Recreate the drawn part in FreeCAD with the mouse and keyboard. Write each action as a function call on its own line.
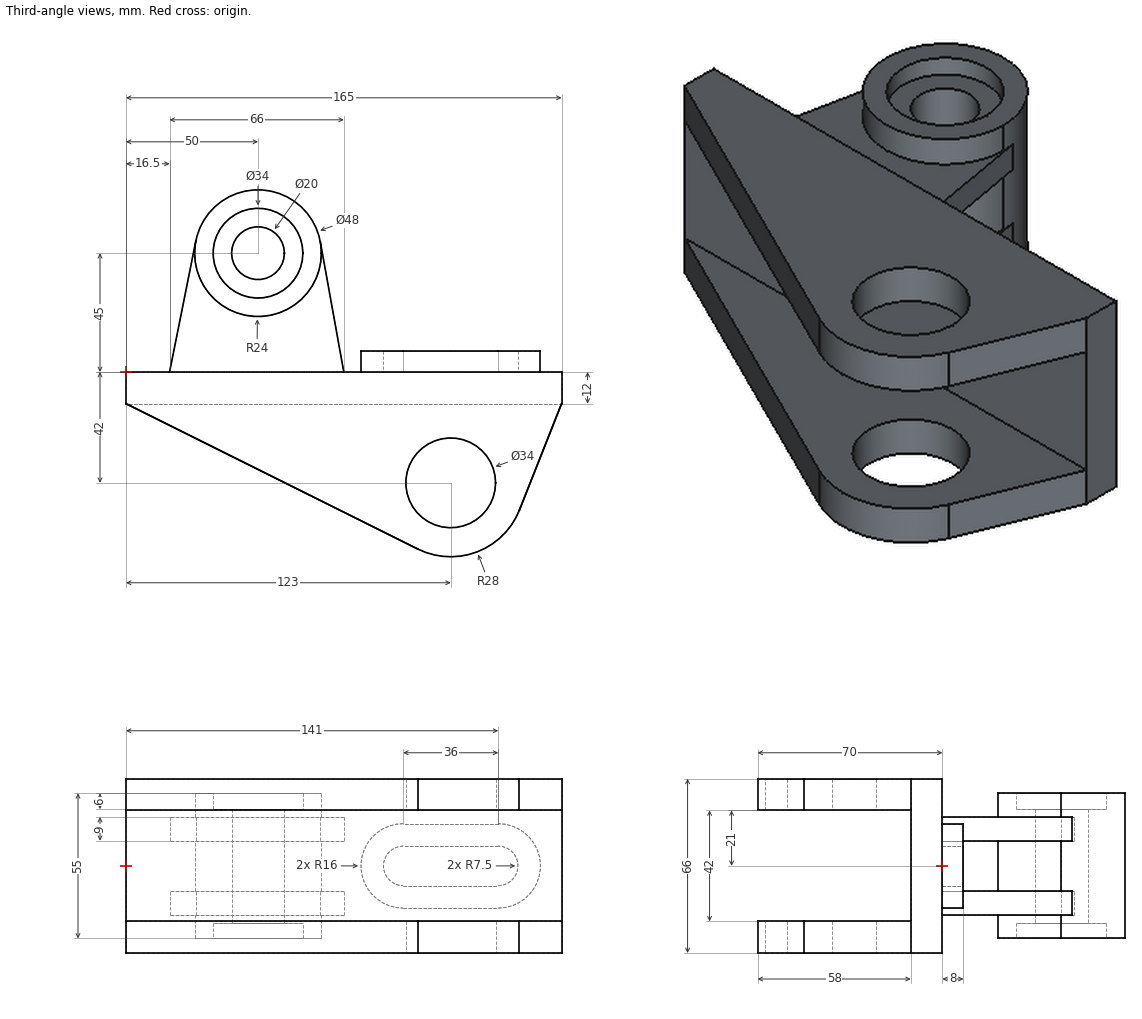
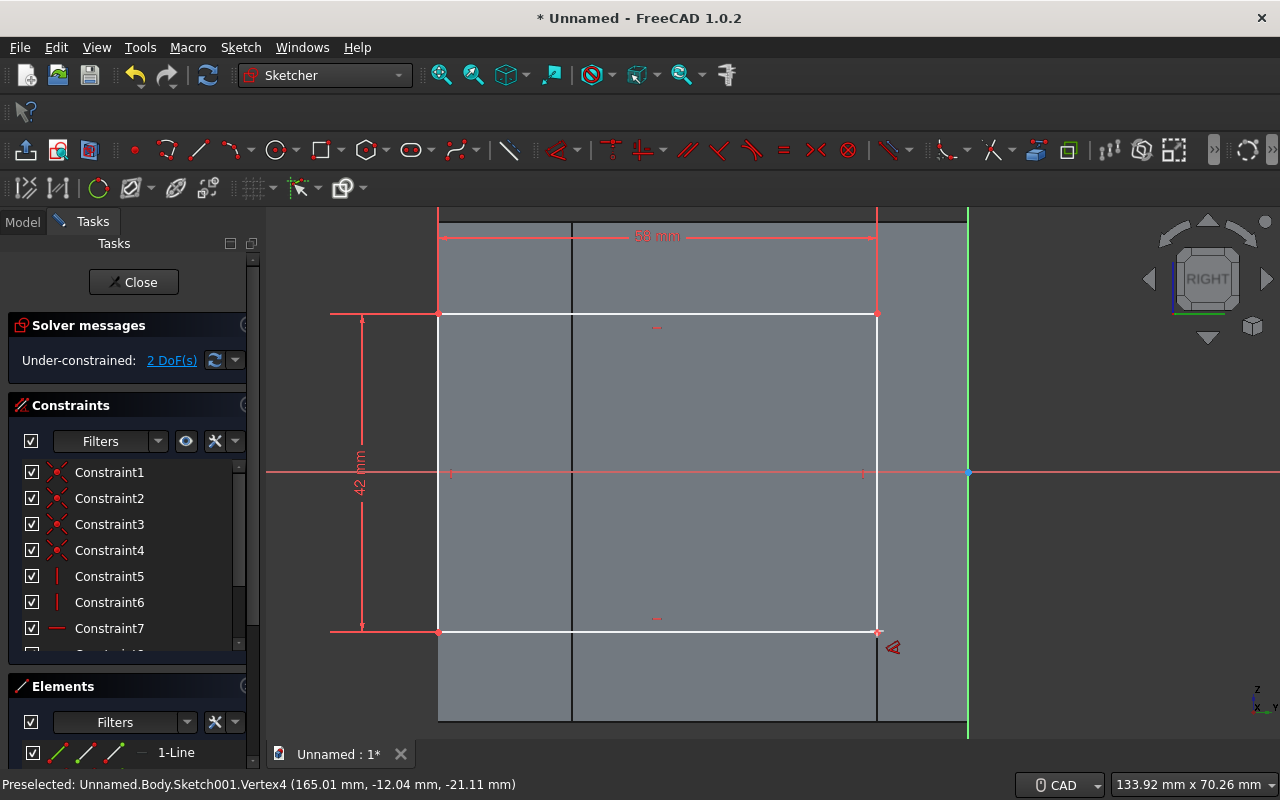
click(438, 314)
click(703, 280)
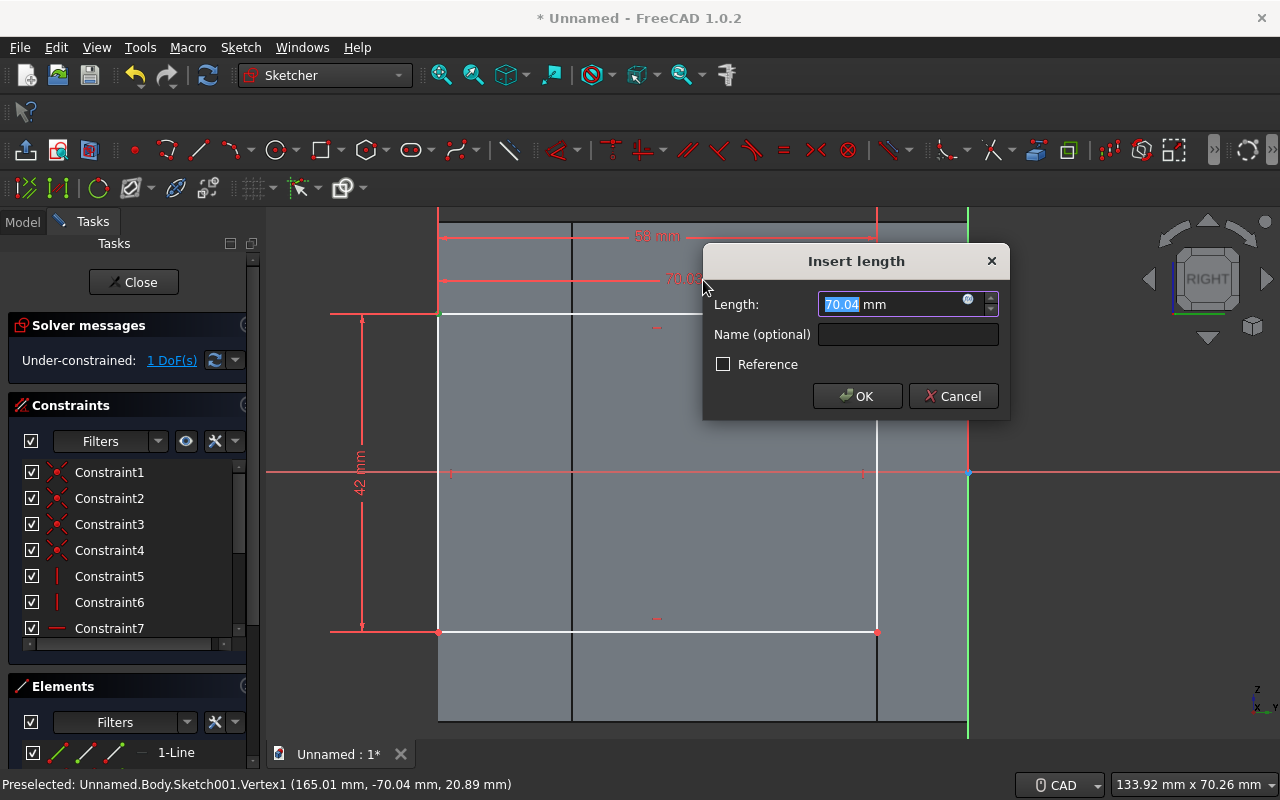
text(70)
key(Return)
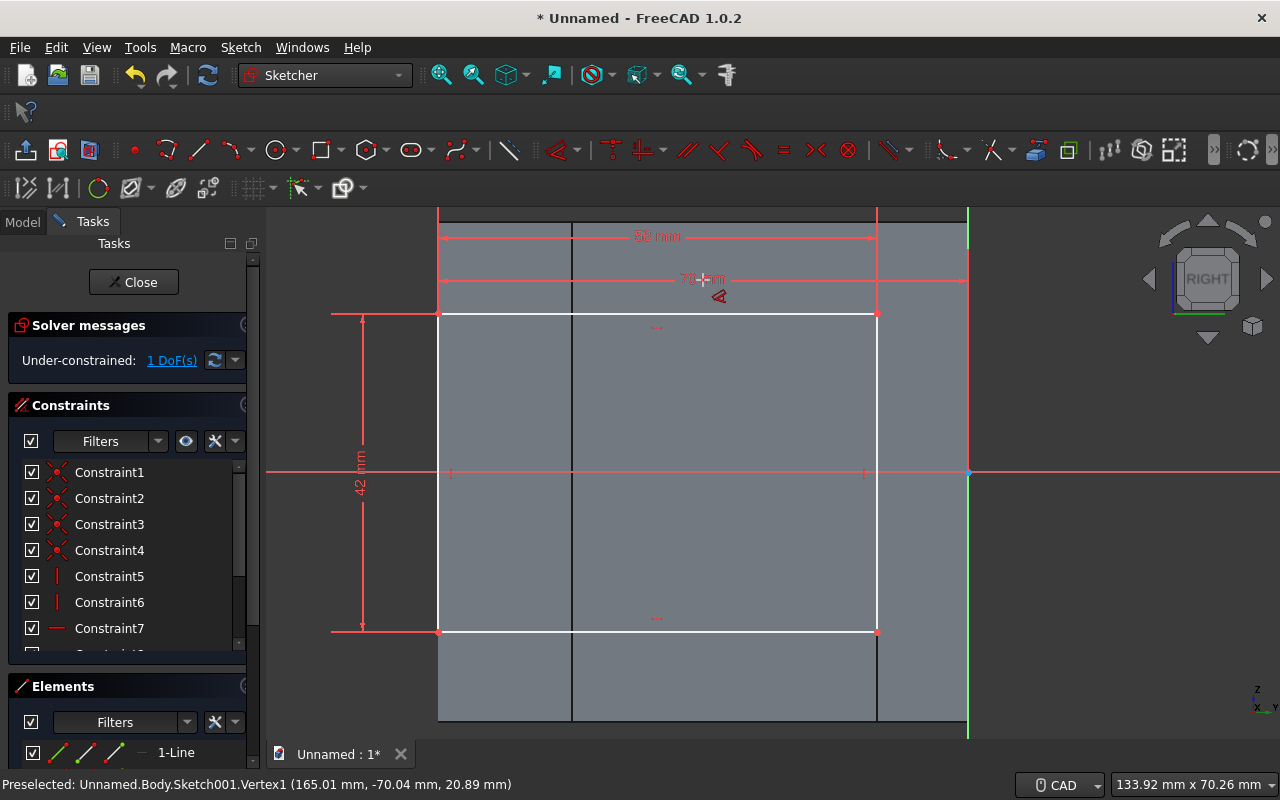
click(438, 314)
click(1002, 393)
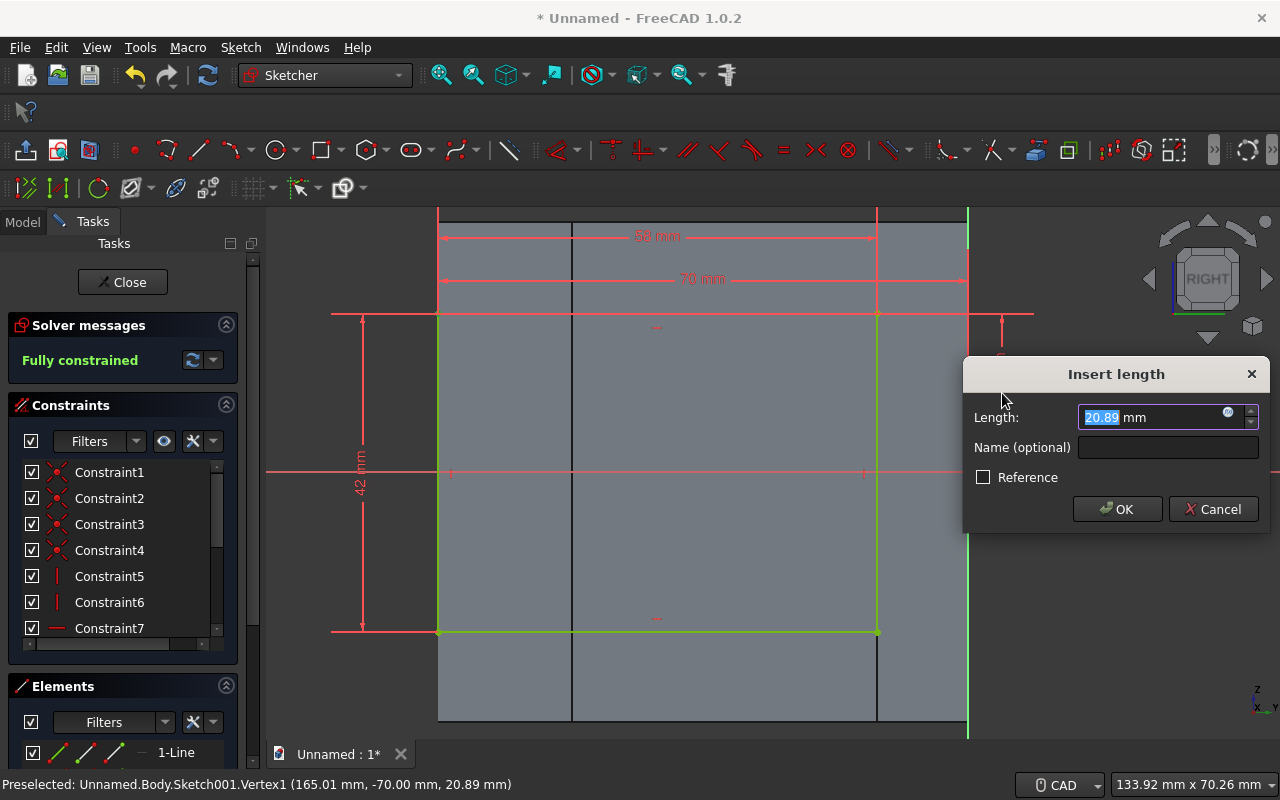
text(21)
key(Return)
key(Escape)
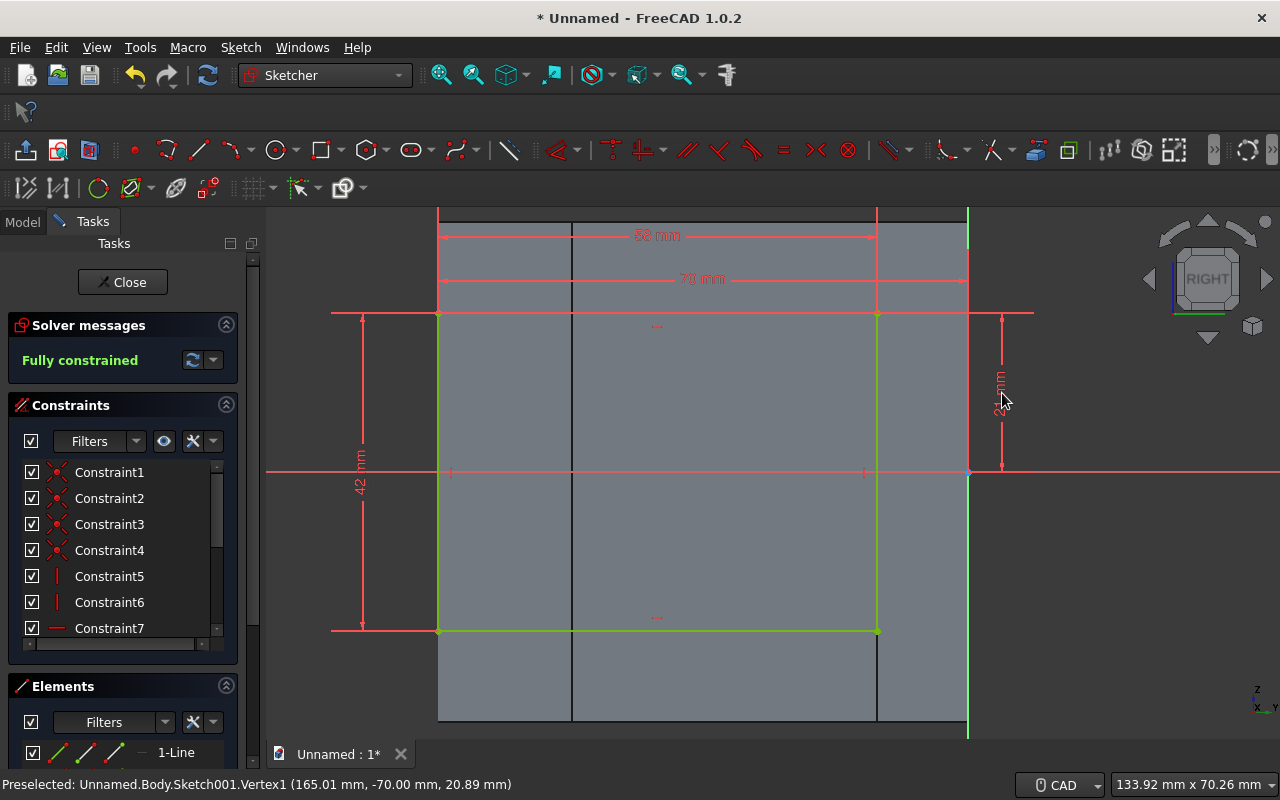
click(123, 282)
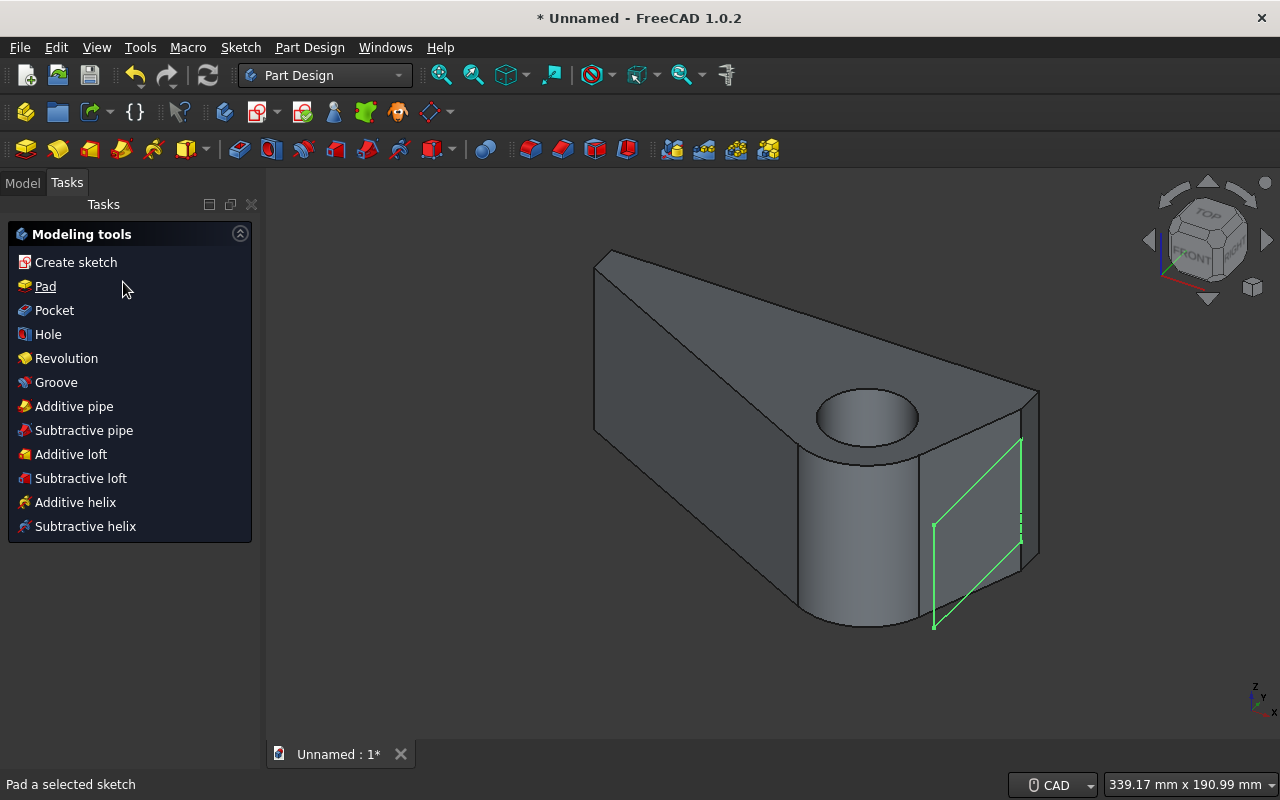
click(240, 150)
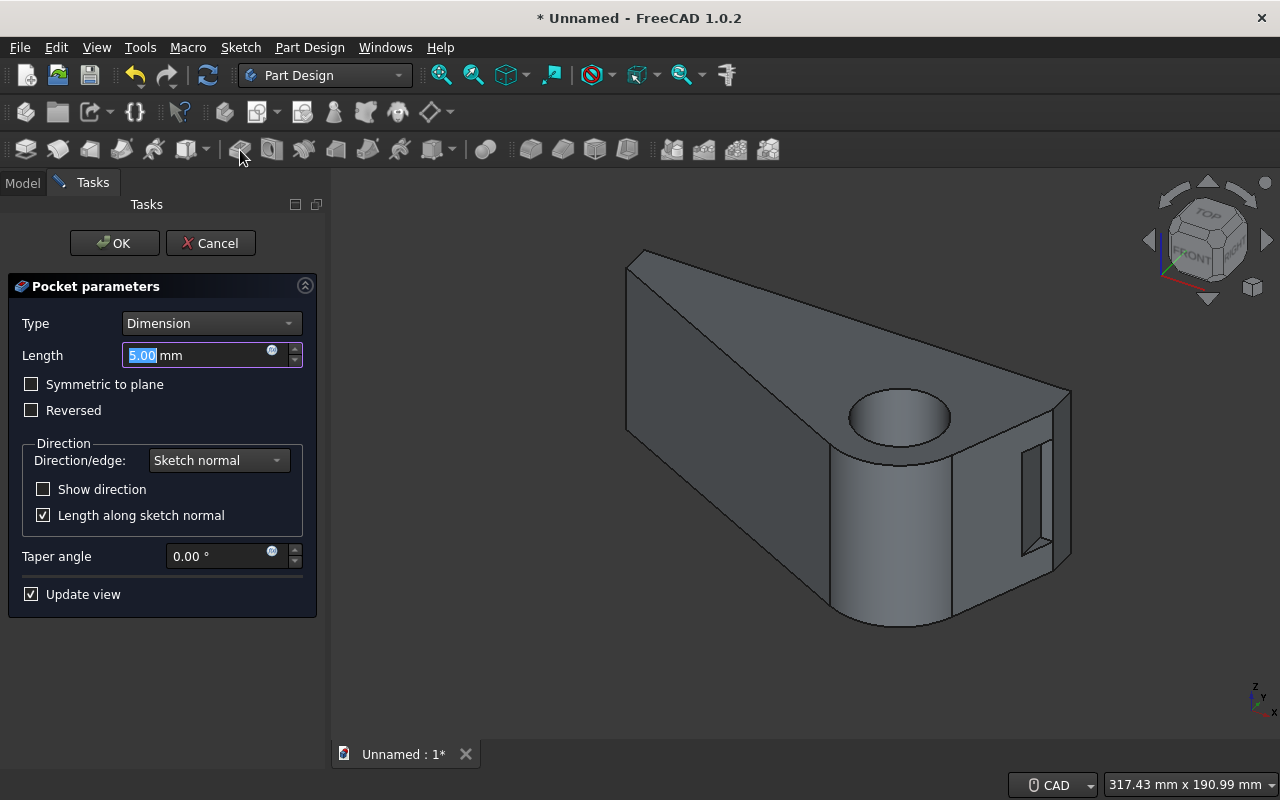
click(212, 324)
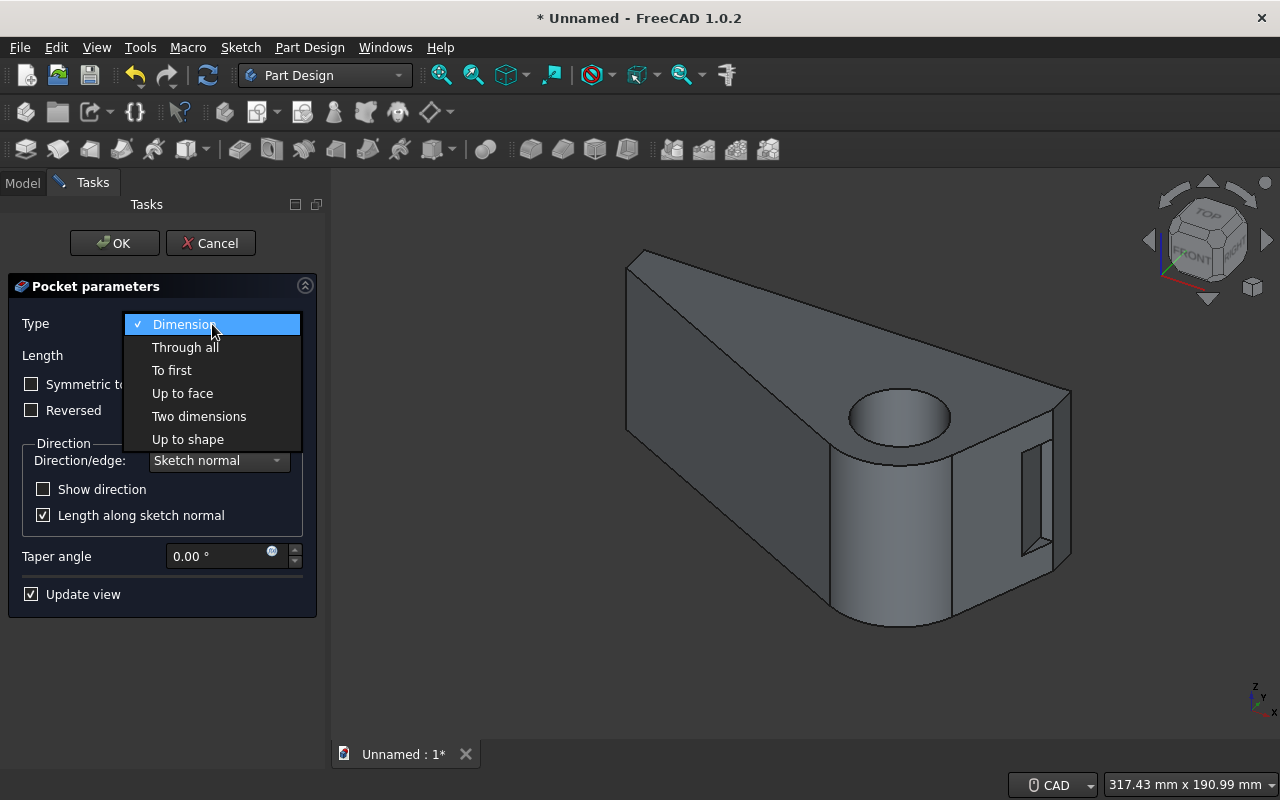
click(212, 348)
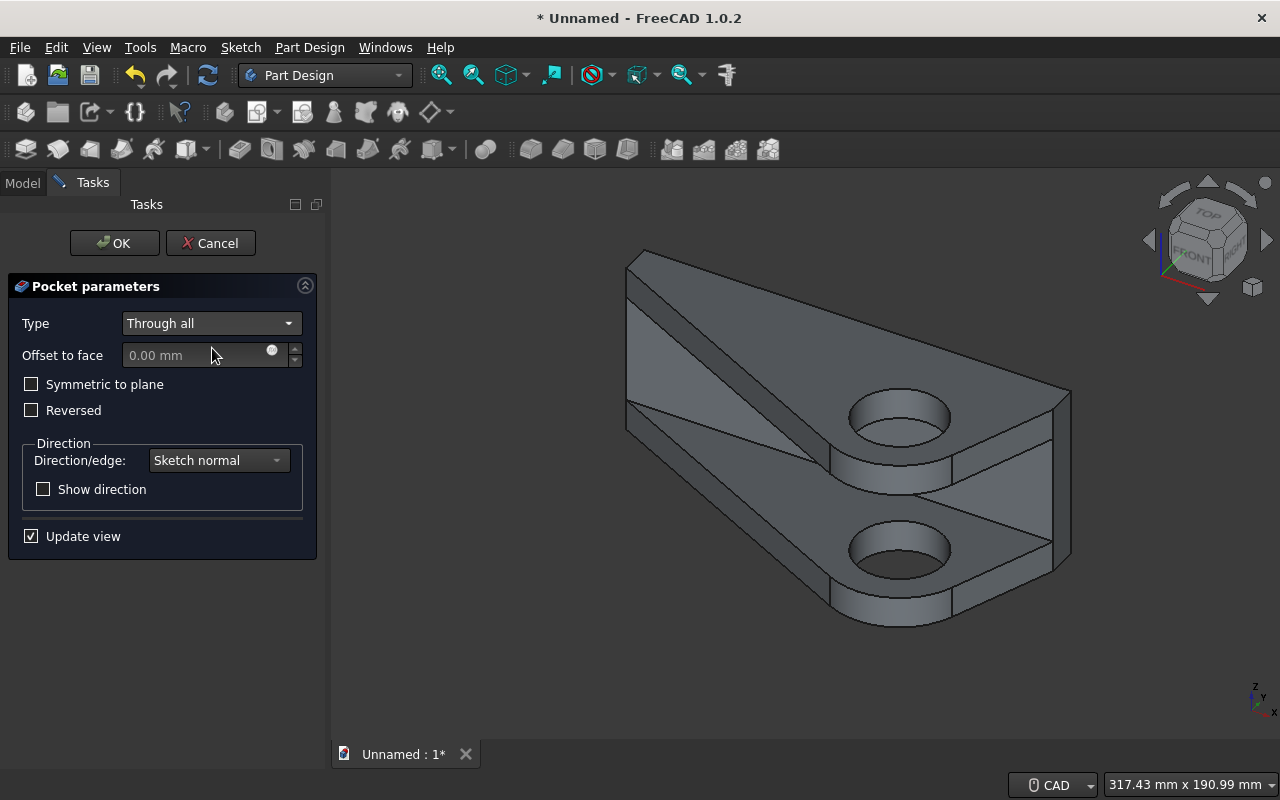
click(115, 243)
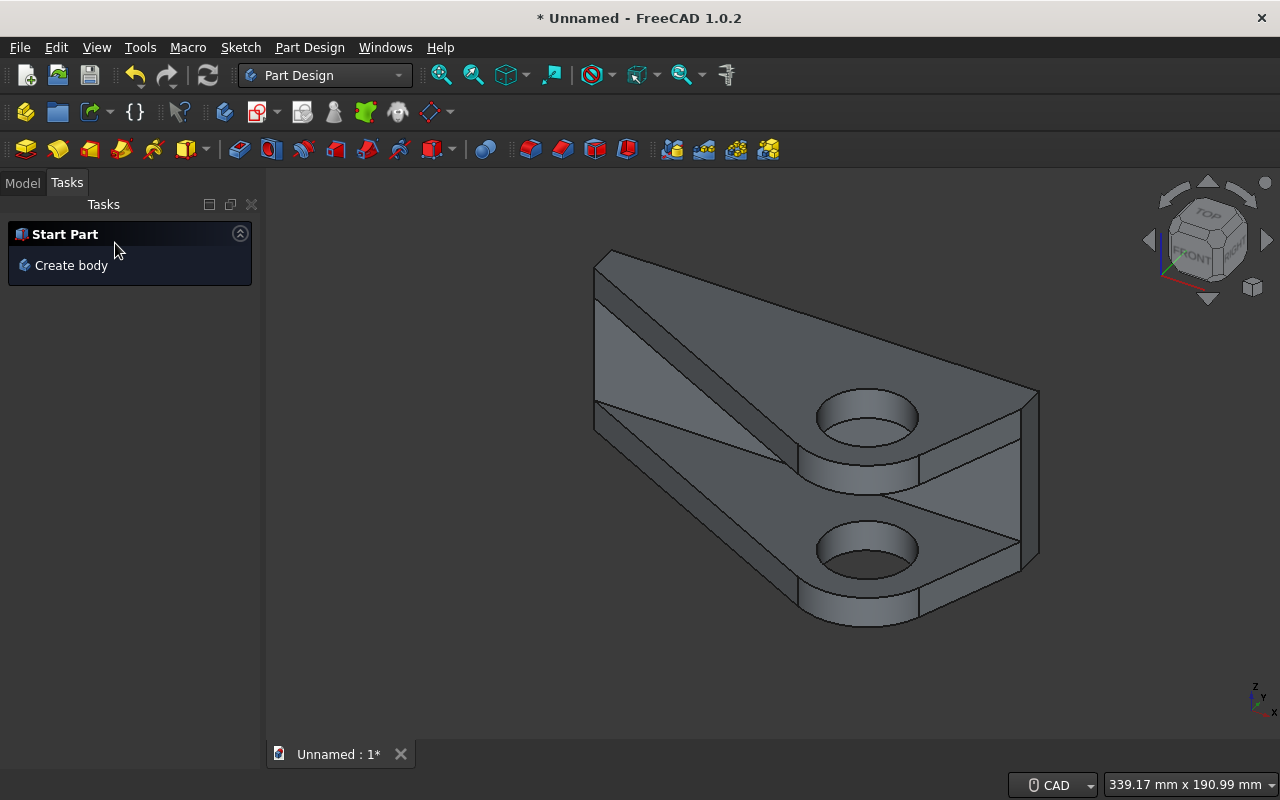
key(4)